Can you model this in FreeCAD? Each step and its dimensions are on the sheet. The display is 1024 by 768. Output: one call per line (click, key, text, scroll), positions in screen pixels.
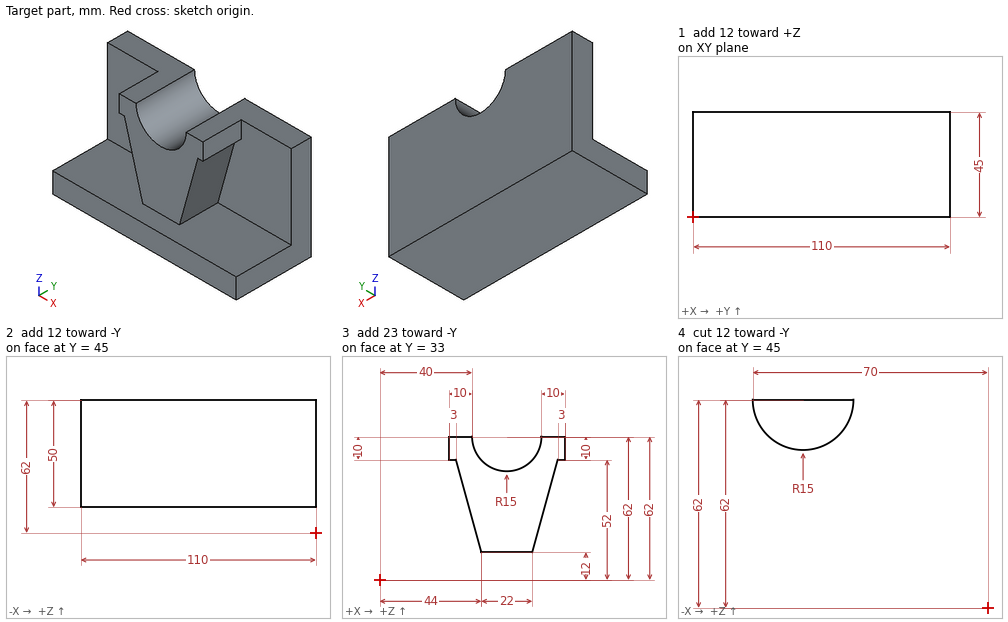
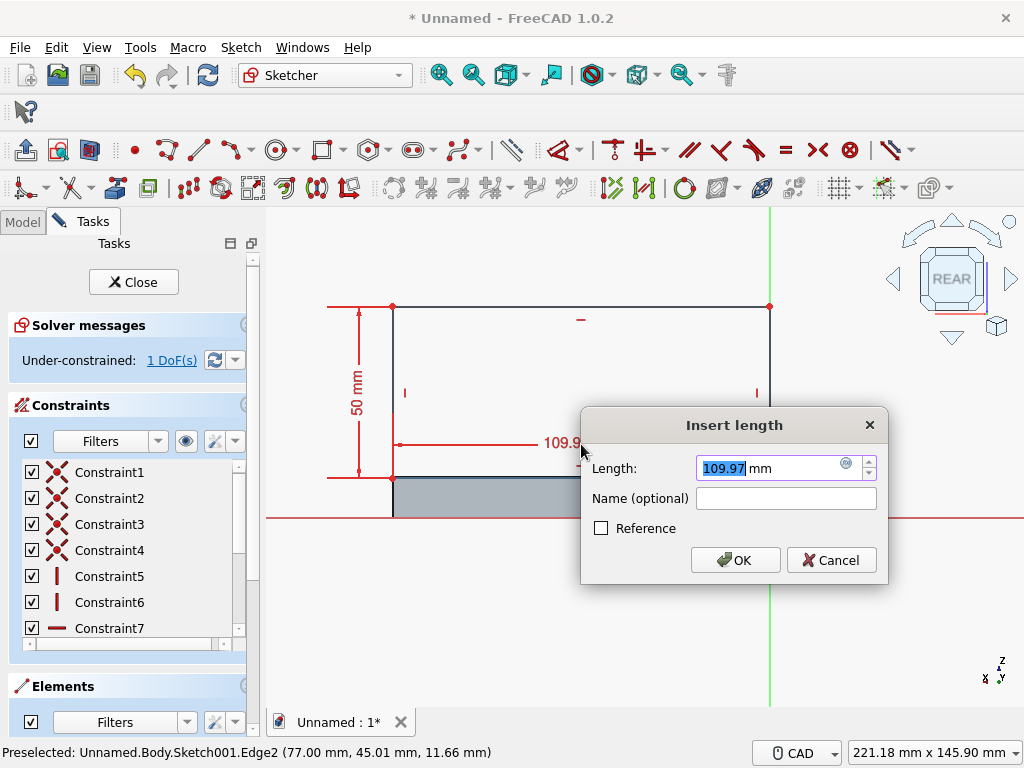
text(110)
key(Return)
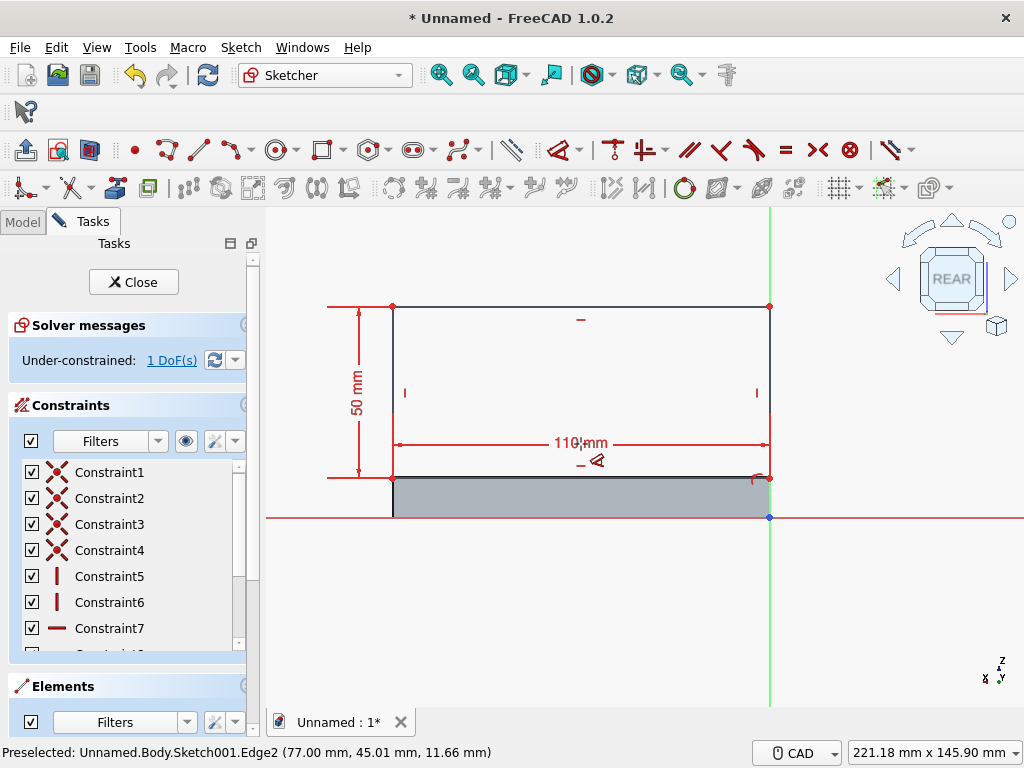
click(393, 307)
click(804, 412)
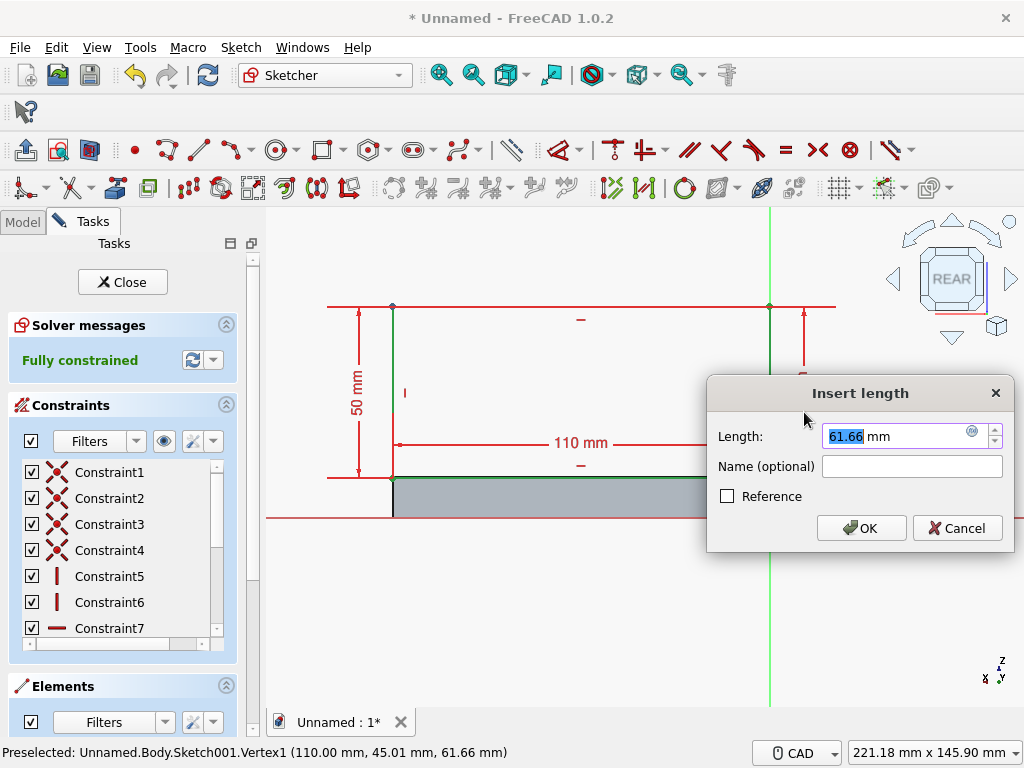
text(62)
key(Return)
key(Escape)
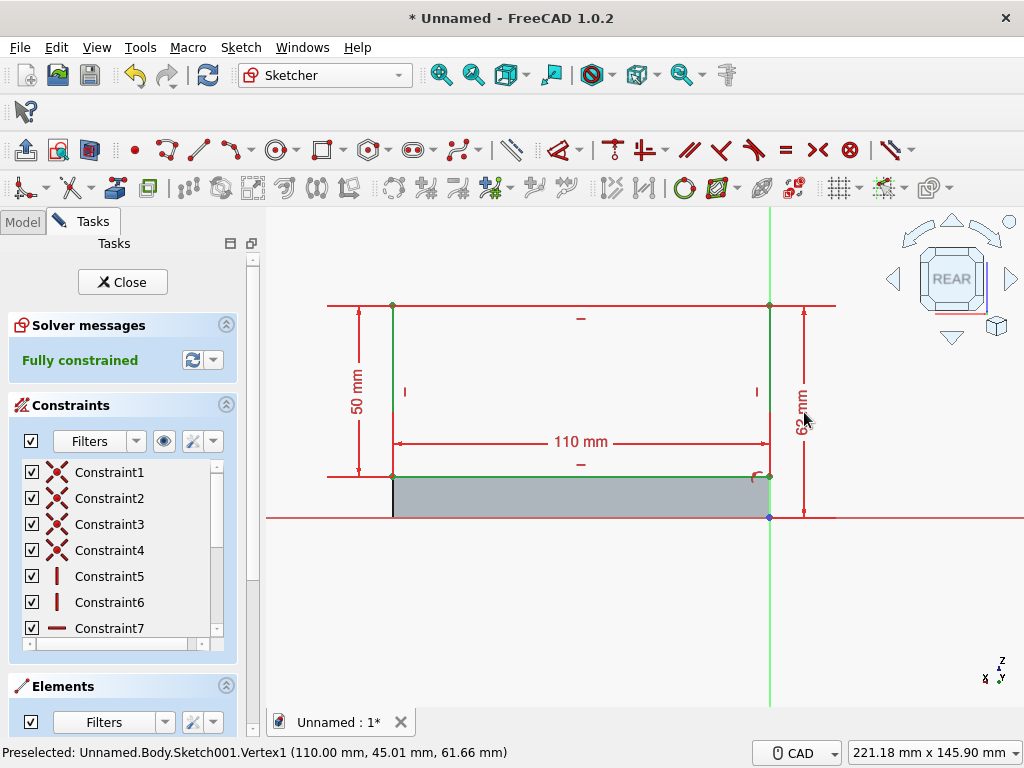
click(123, 282)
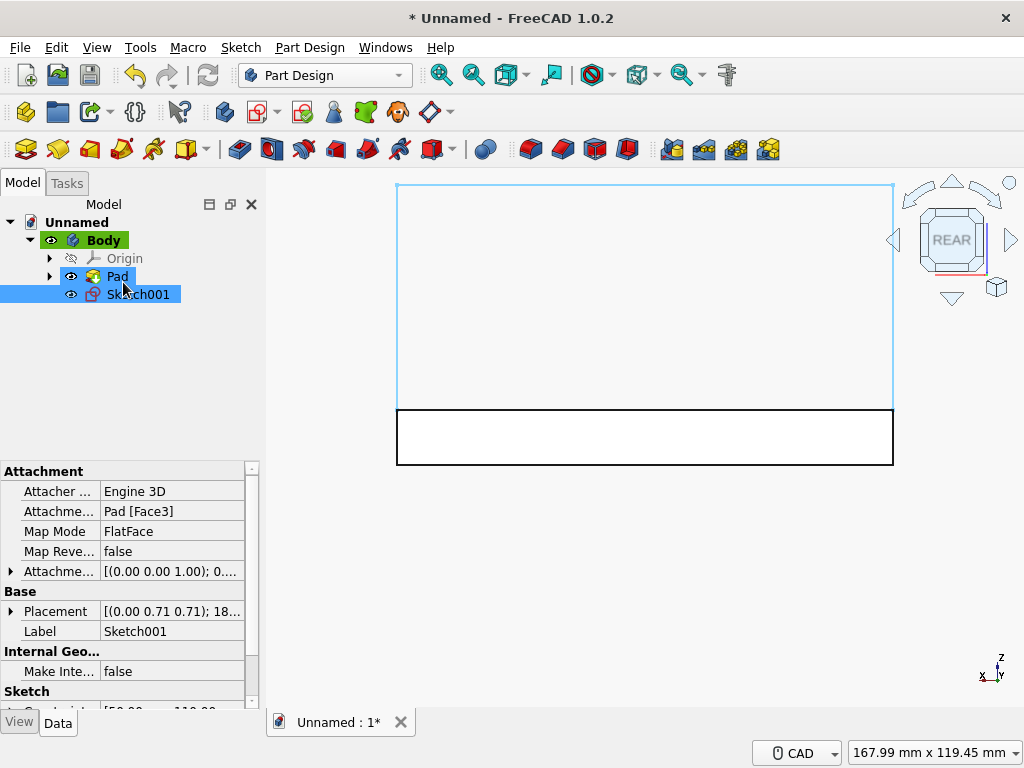
click(26, 150)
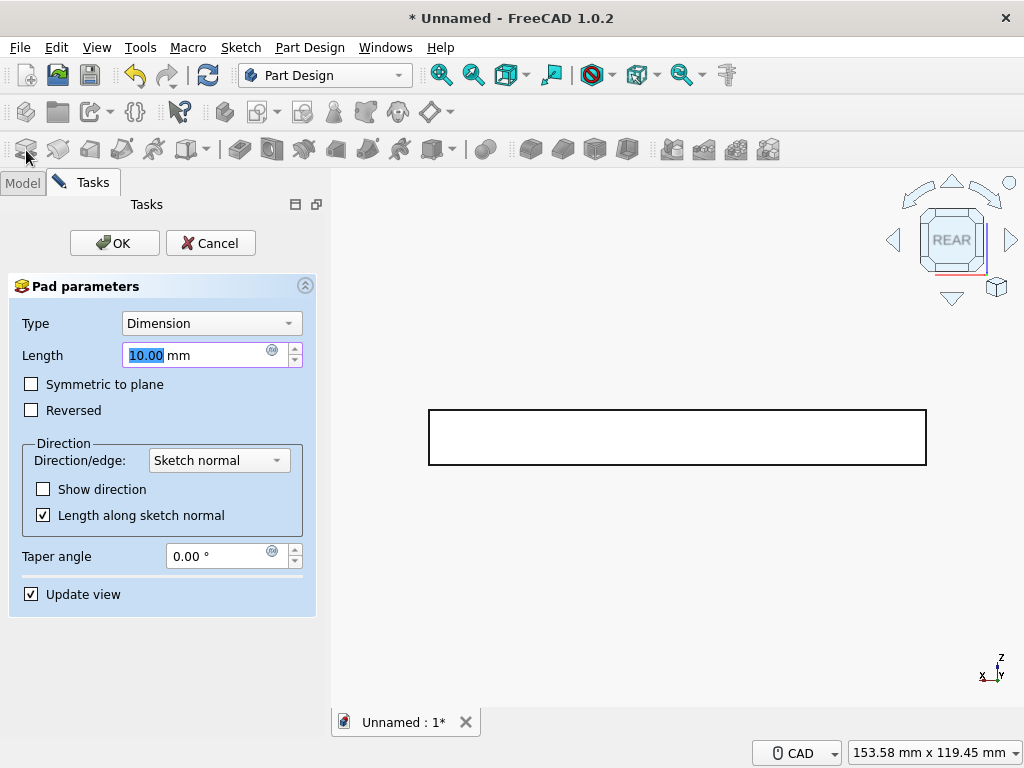
text(12)
key(Tab)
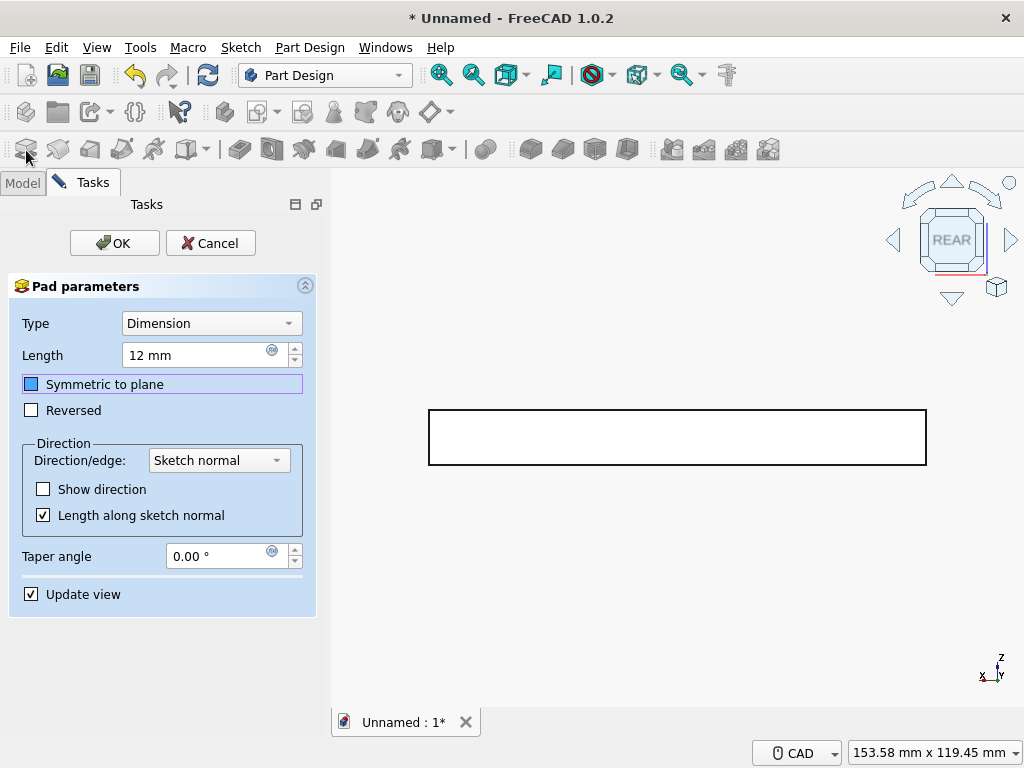
click(30, 410)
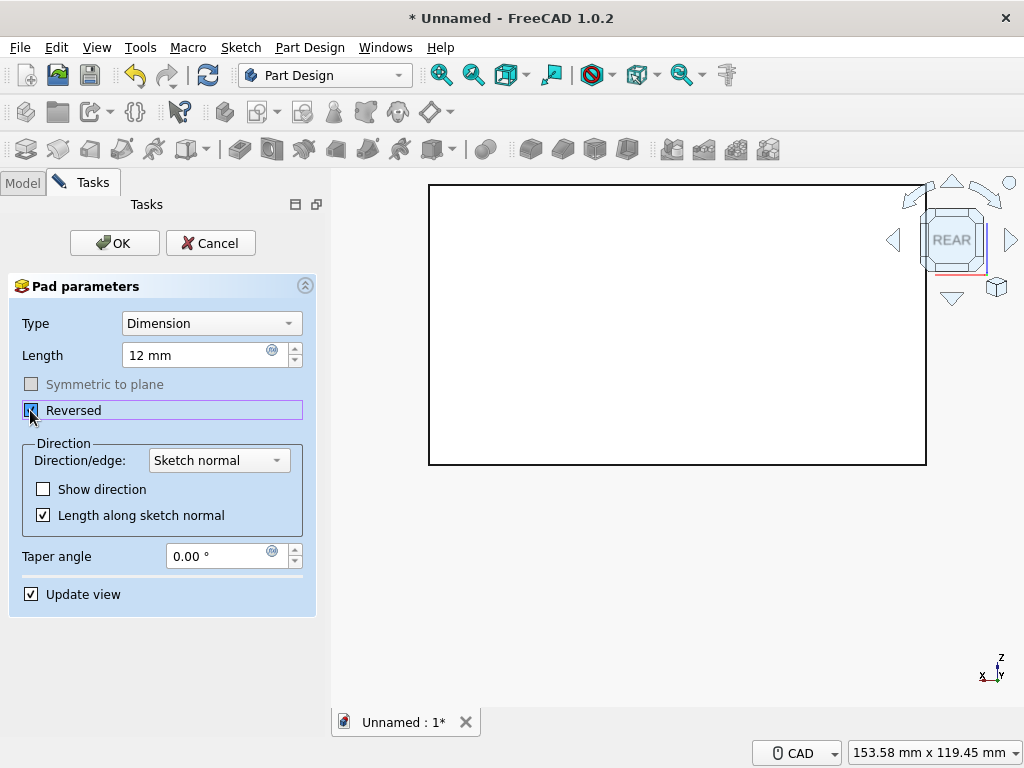
click(115, 243)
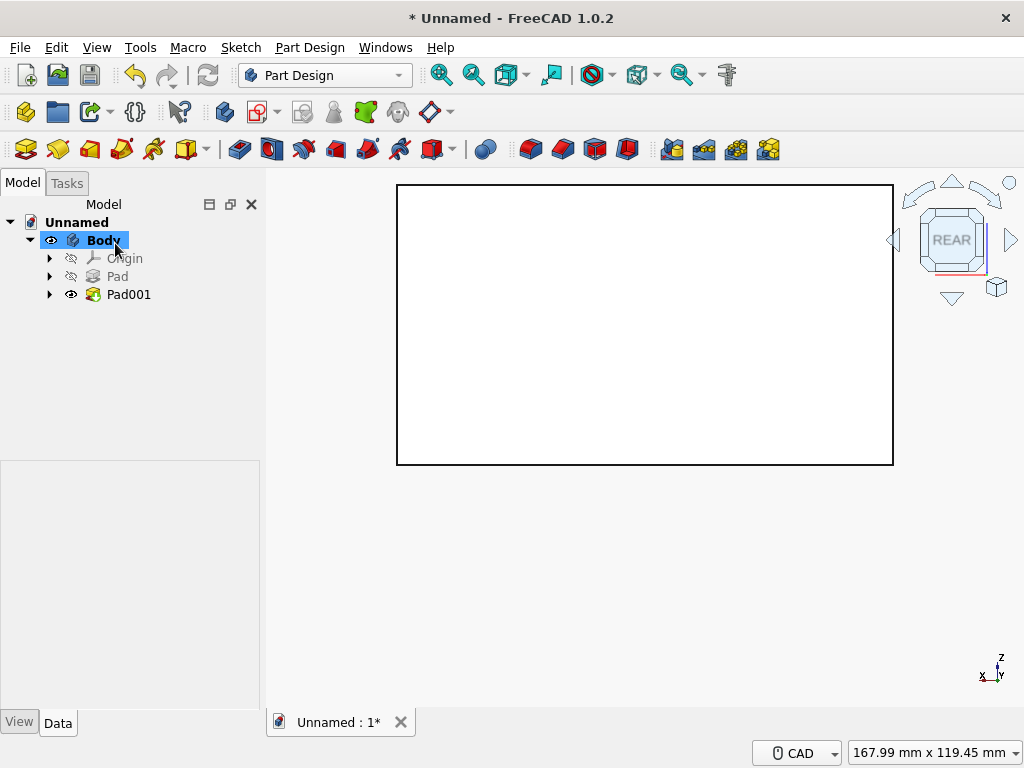
key(0)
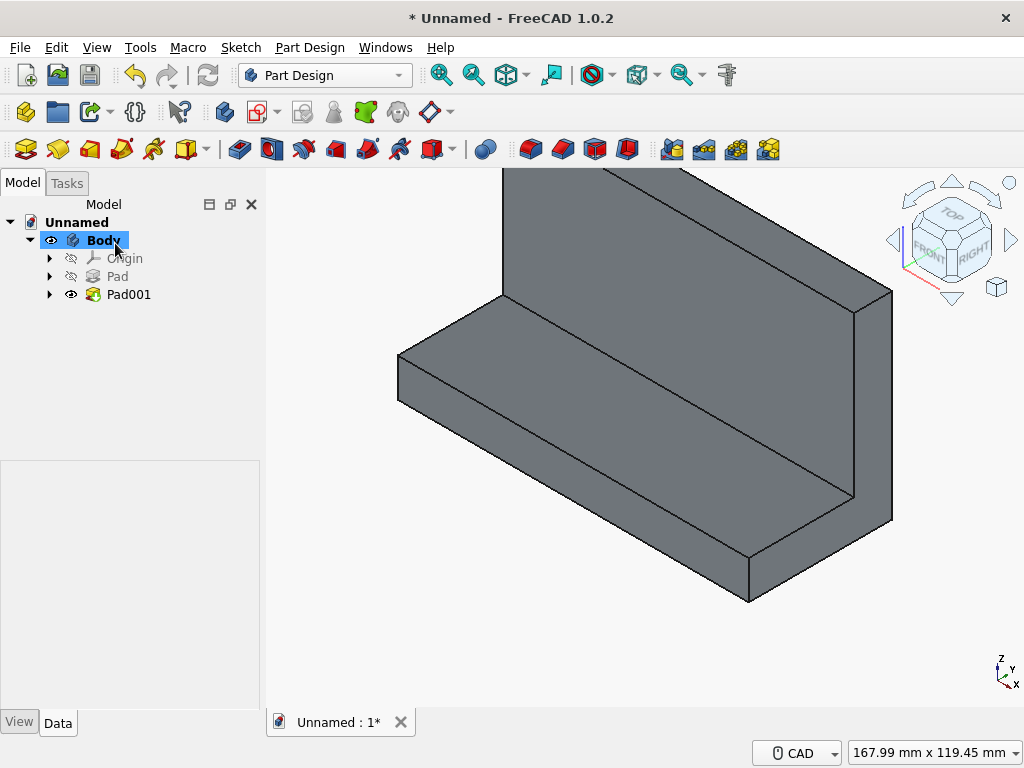
click(442, 76)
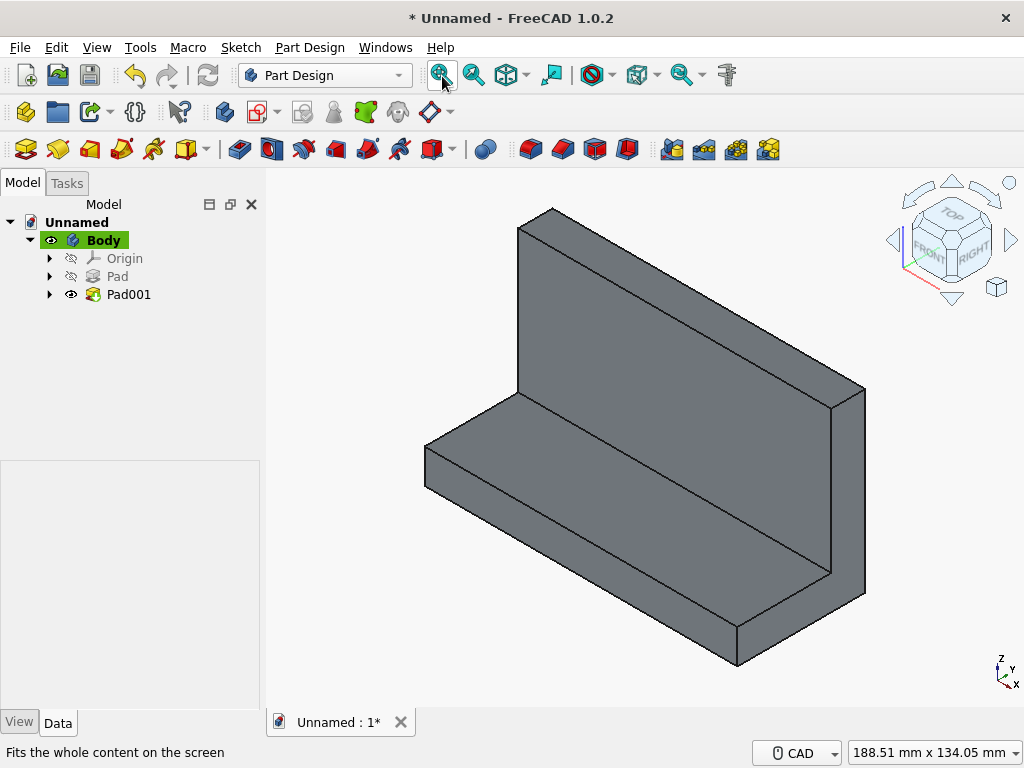
click(720, 425)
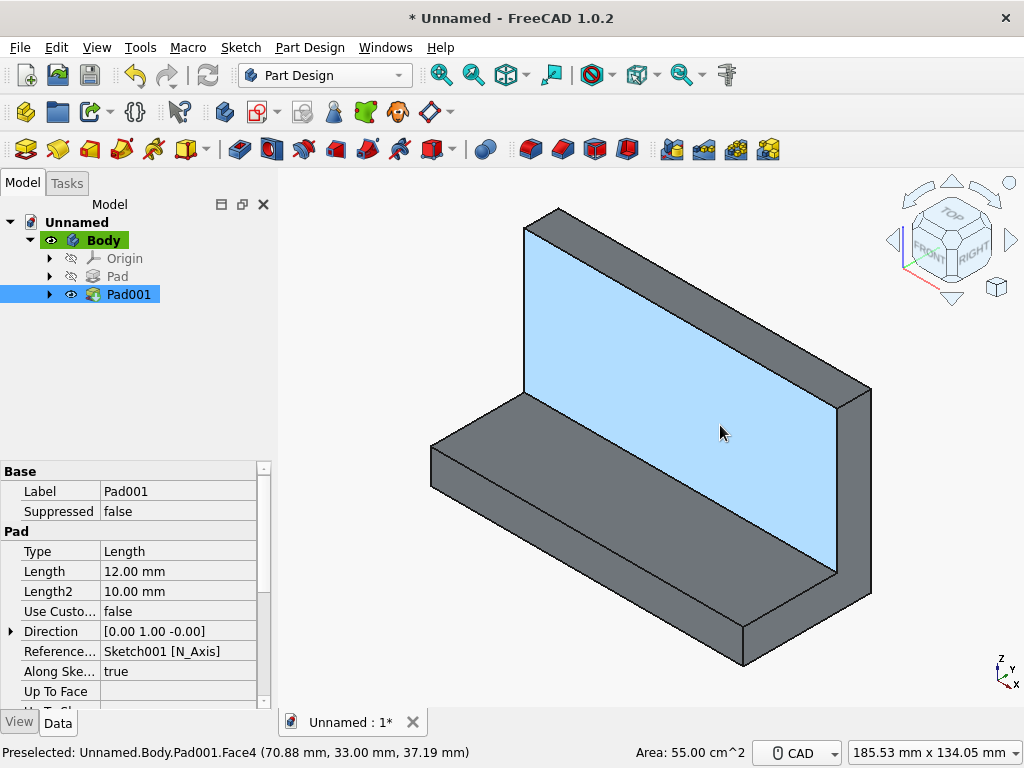
click(258, 112)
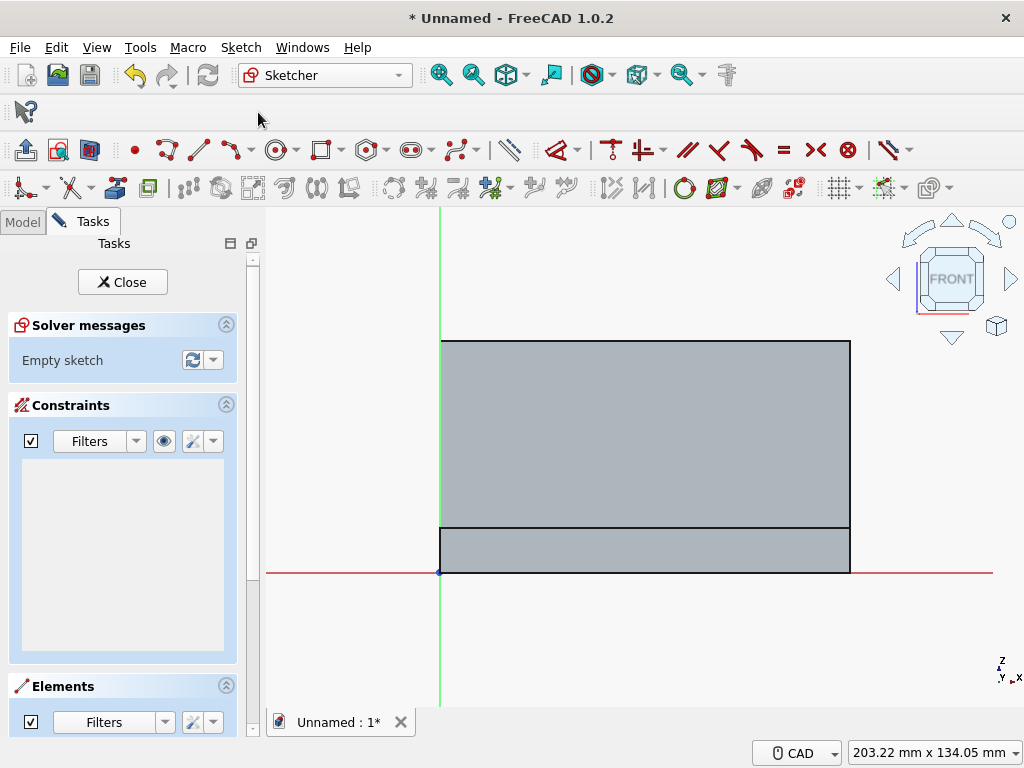
click(90, 150)